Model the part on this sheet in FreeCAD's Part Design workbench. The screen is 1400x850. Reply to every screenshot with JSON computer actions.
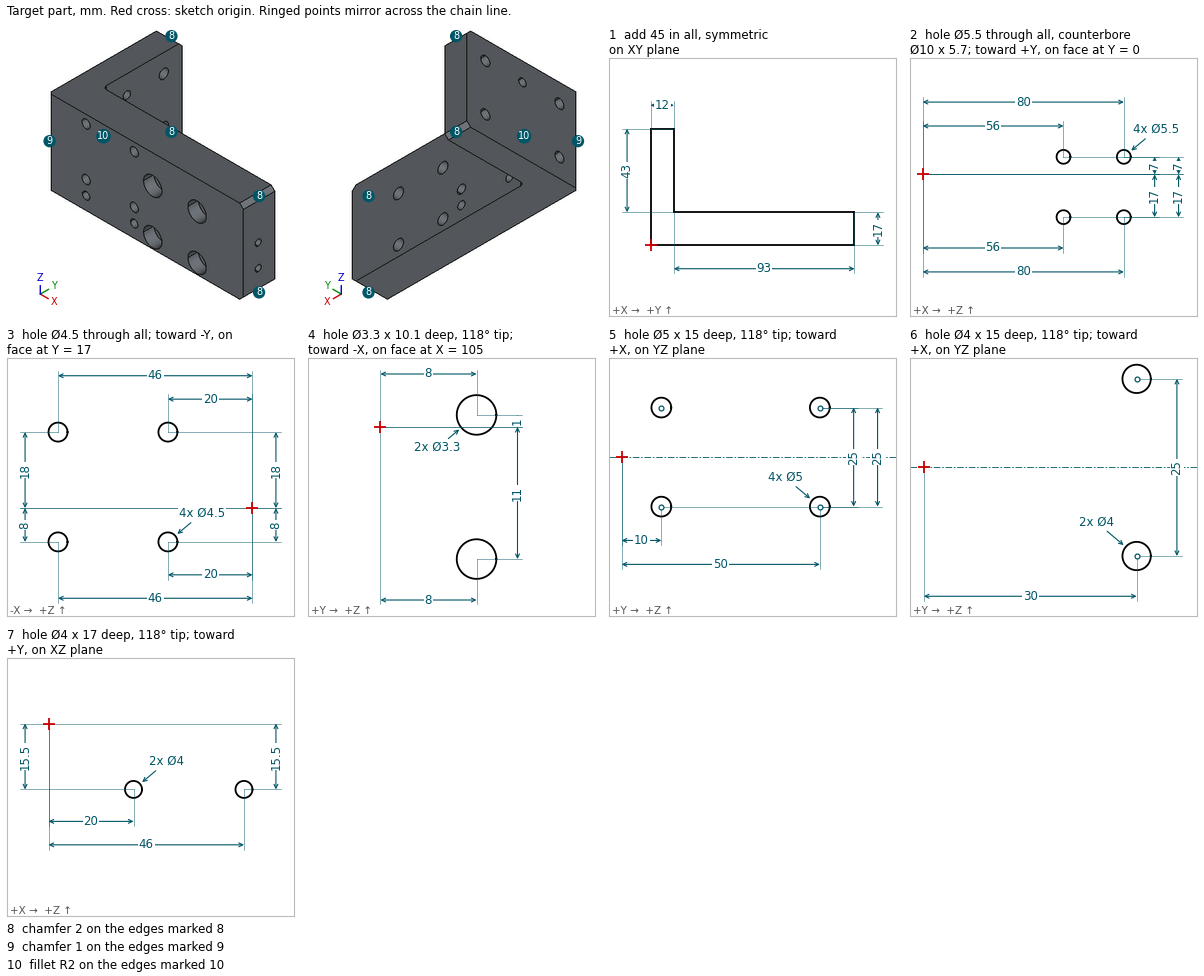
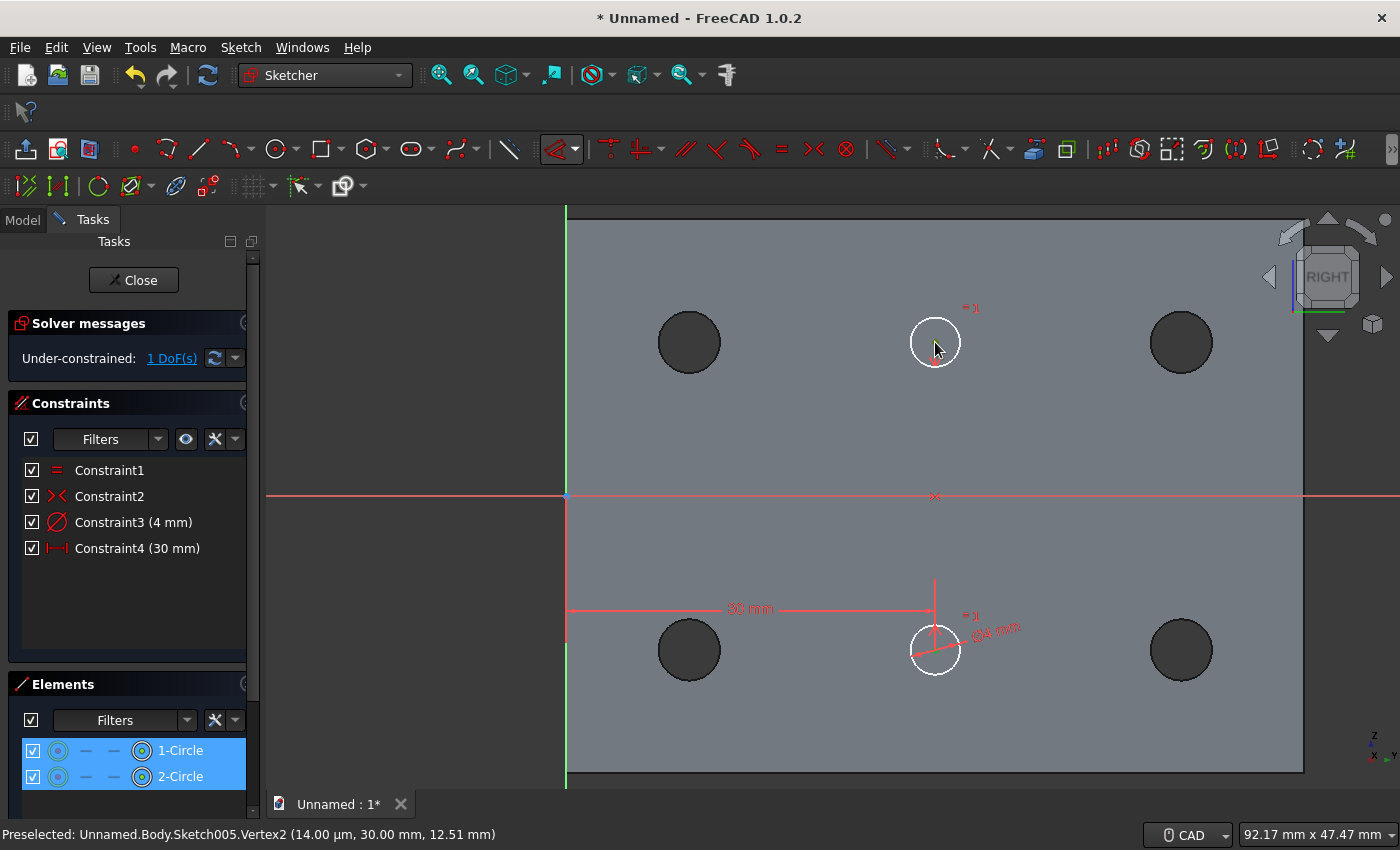
{"action": "key", "text": "i"}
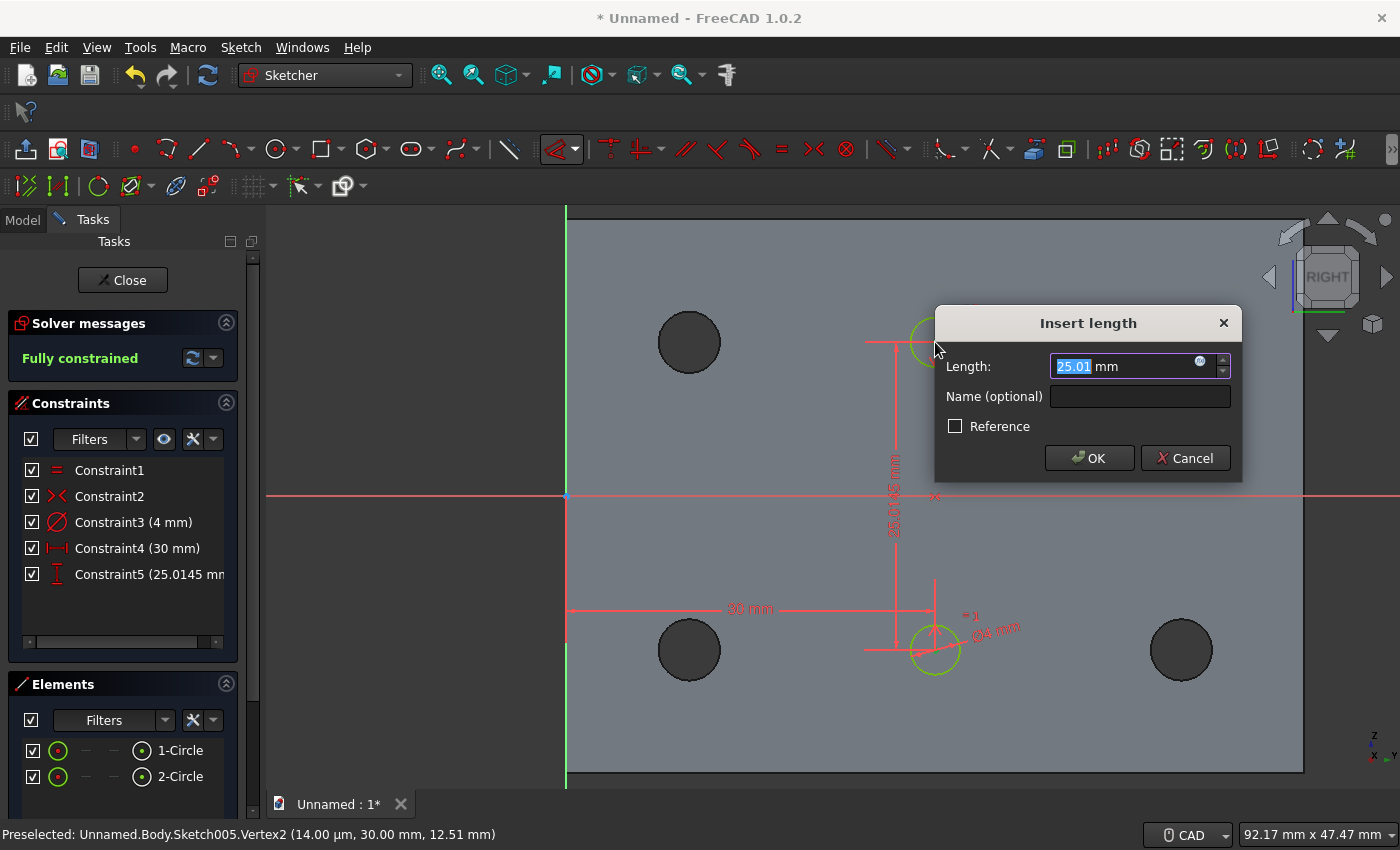
{"action": "type", "text": "25"}
{"action": "key", "text": "Return"}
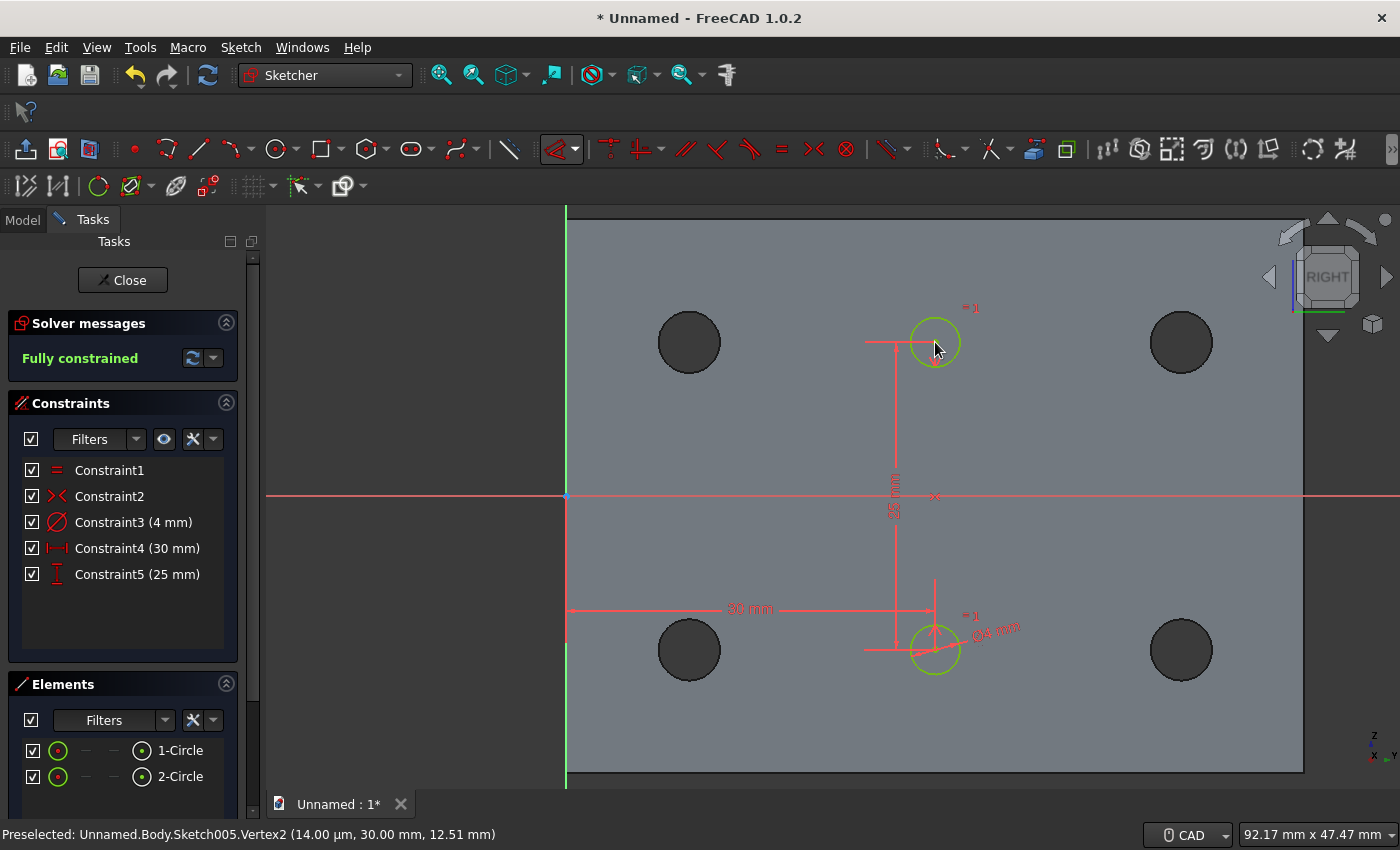
{"action": "left_click", "coordinate": [123, 280]}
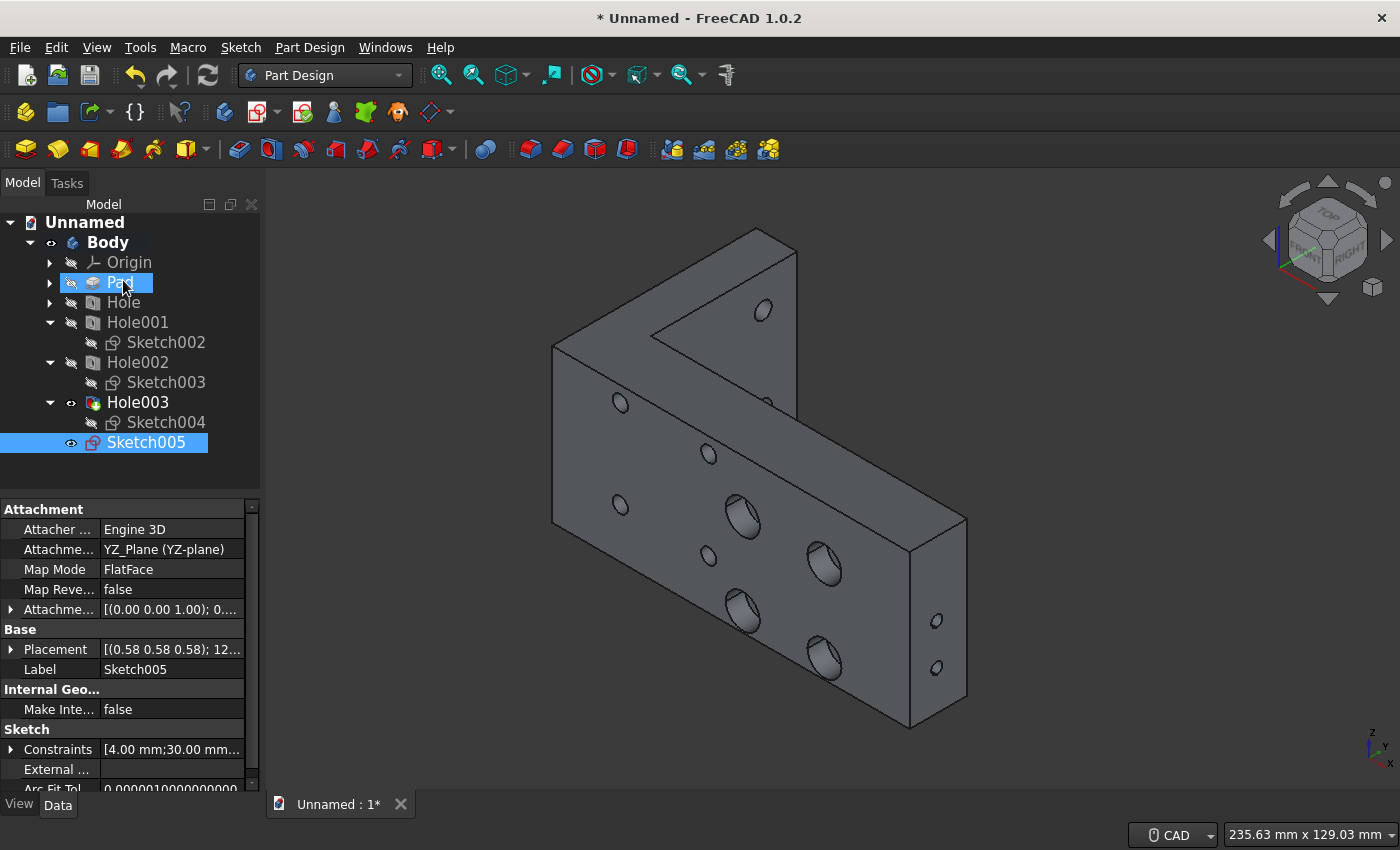
{"action": "left_click", "coordinate": [272, 150]}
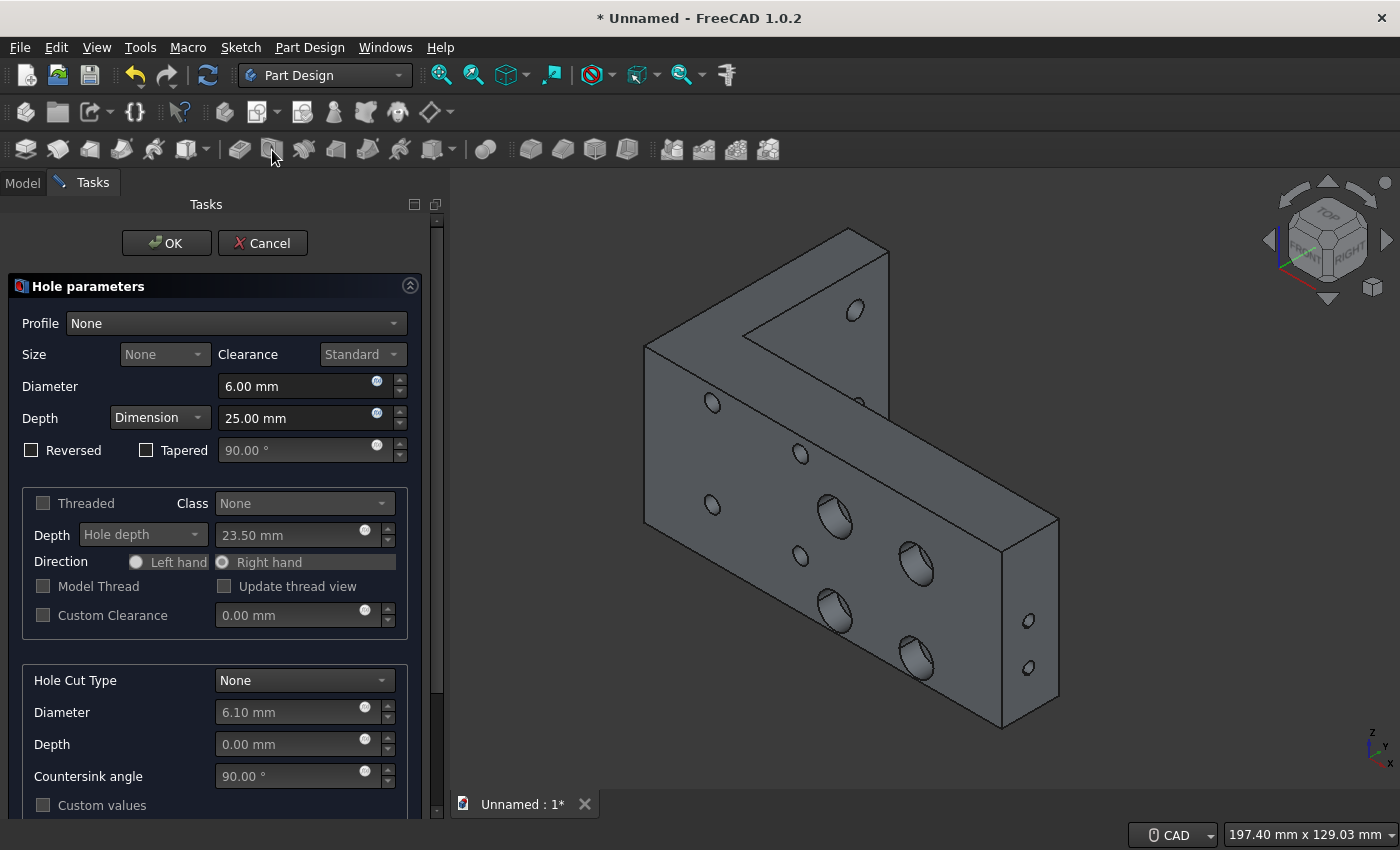
{"action": "triple_click", "coordinate": [305, 386]}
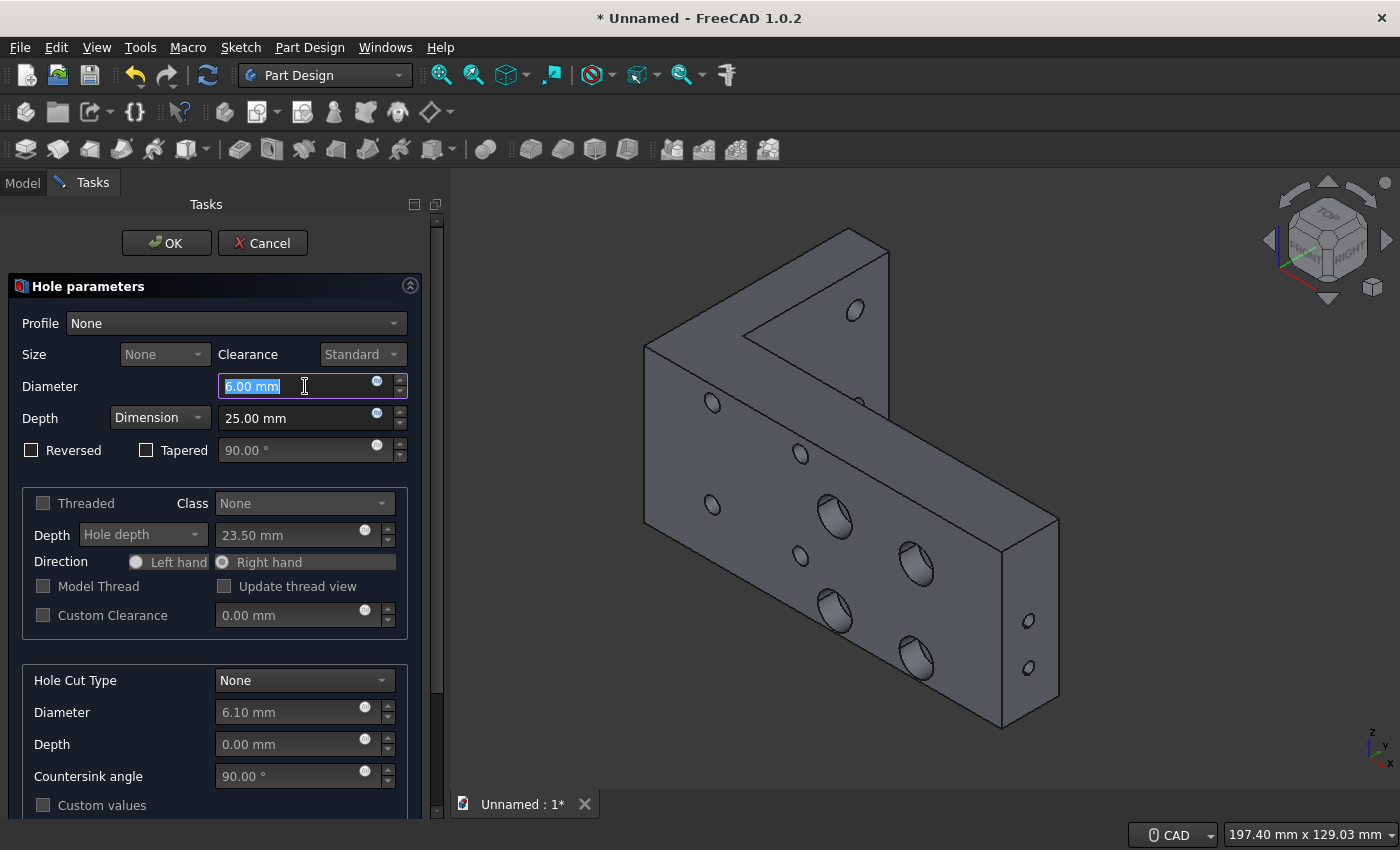
{"action": "type", "text": "4"}
{"action": "key", "text": "Tab"}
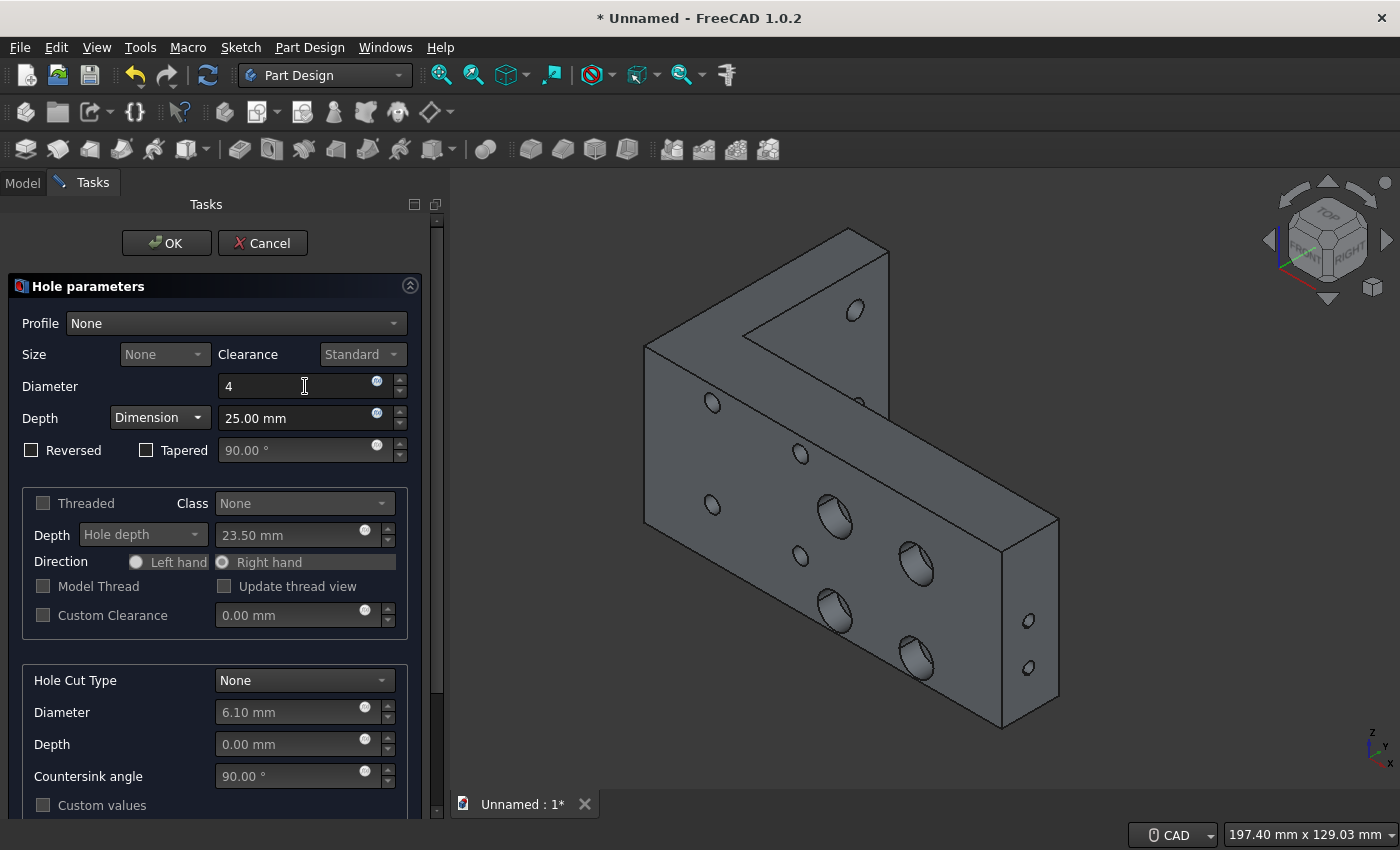
{"action": "triple_click", "coordinate": [305, 418]}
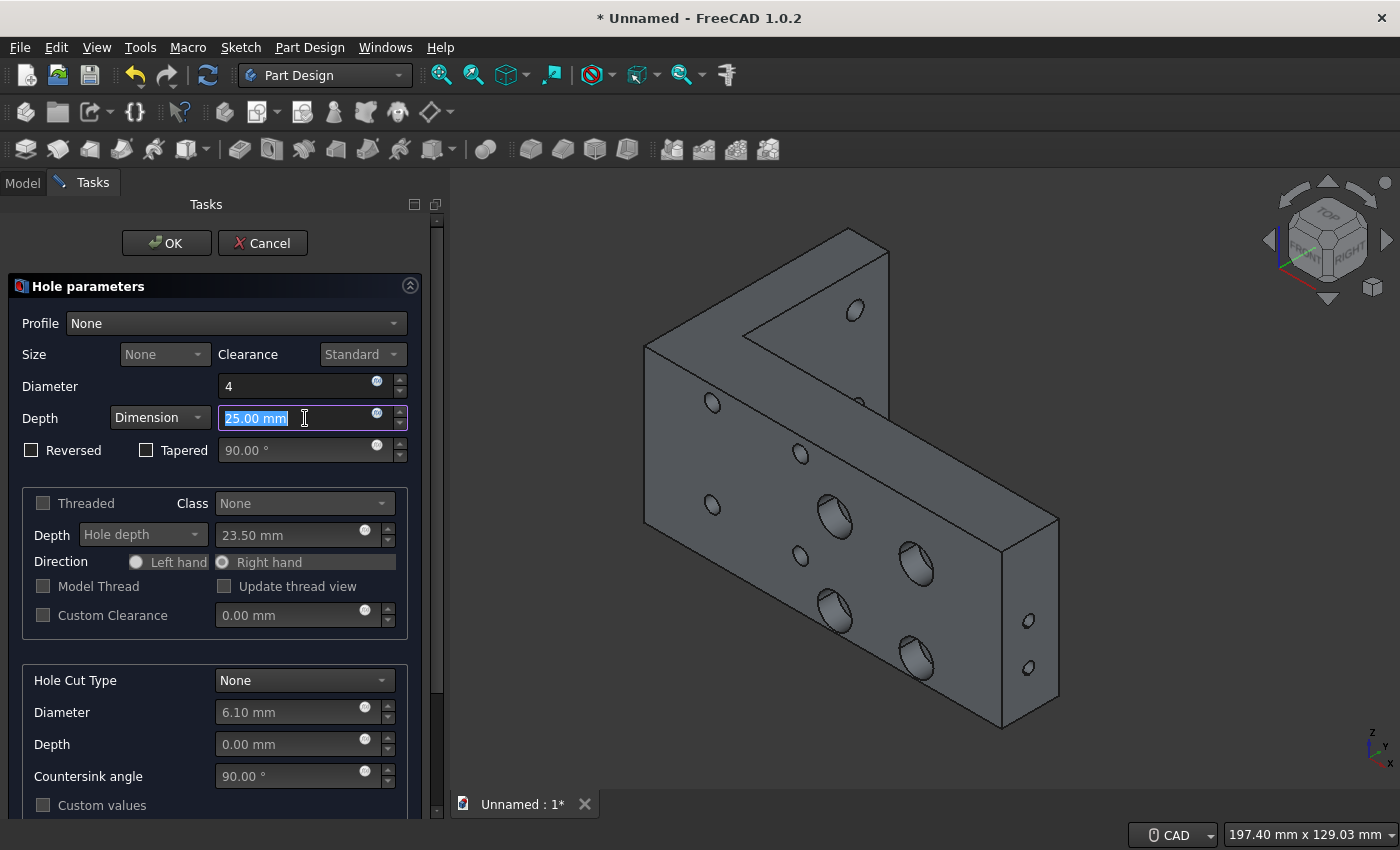
{"action": "type", "text": "15"}
{"action": "key", "text": "Tab"}